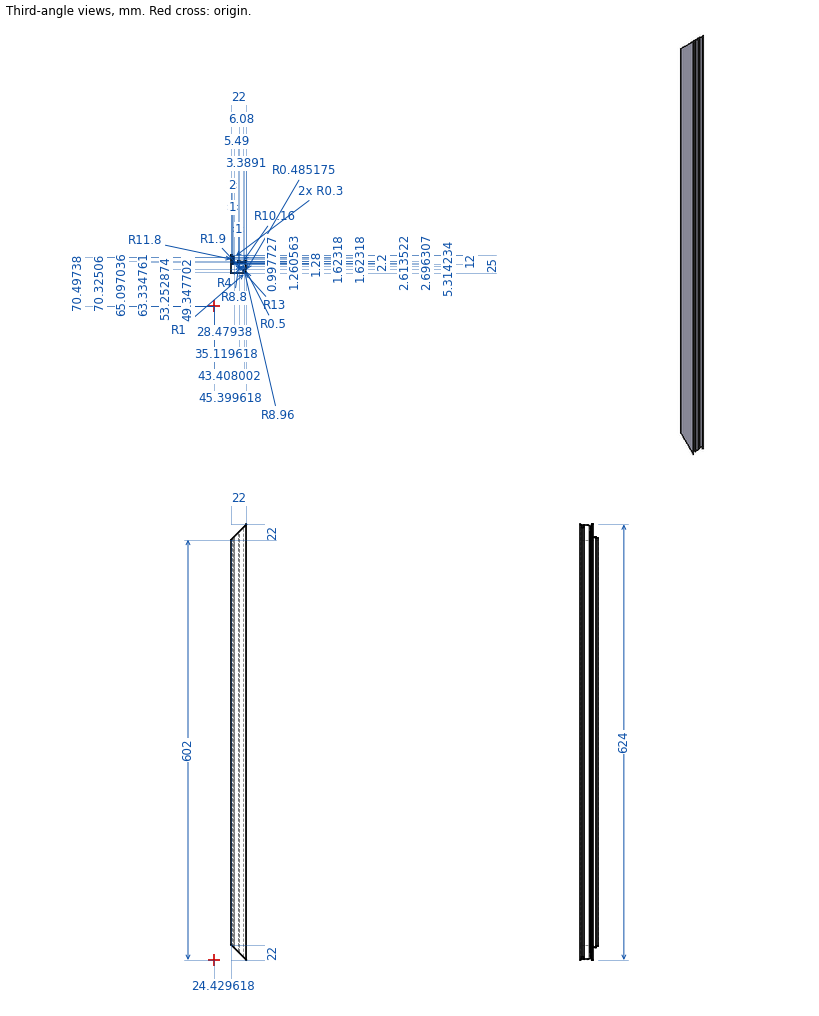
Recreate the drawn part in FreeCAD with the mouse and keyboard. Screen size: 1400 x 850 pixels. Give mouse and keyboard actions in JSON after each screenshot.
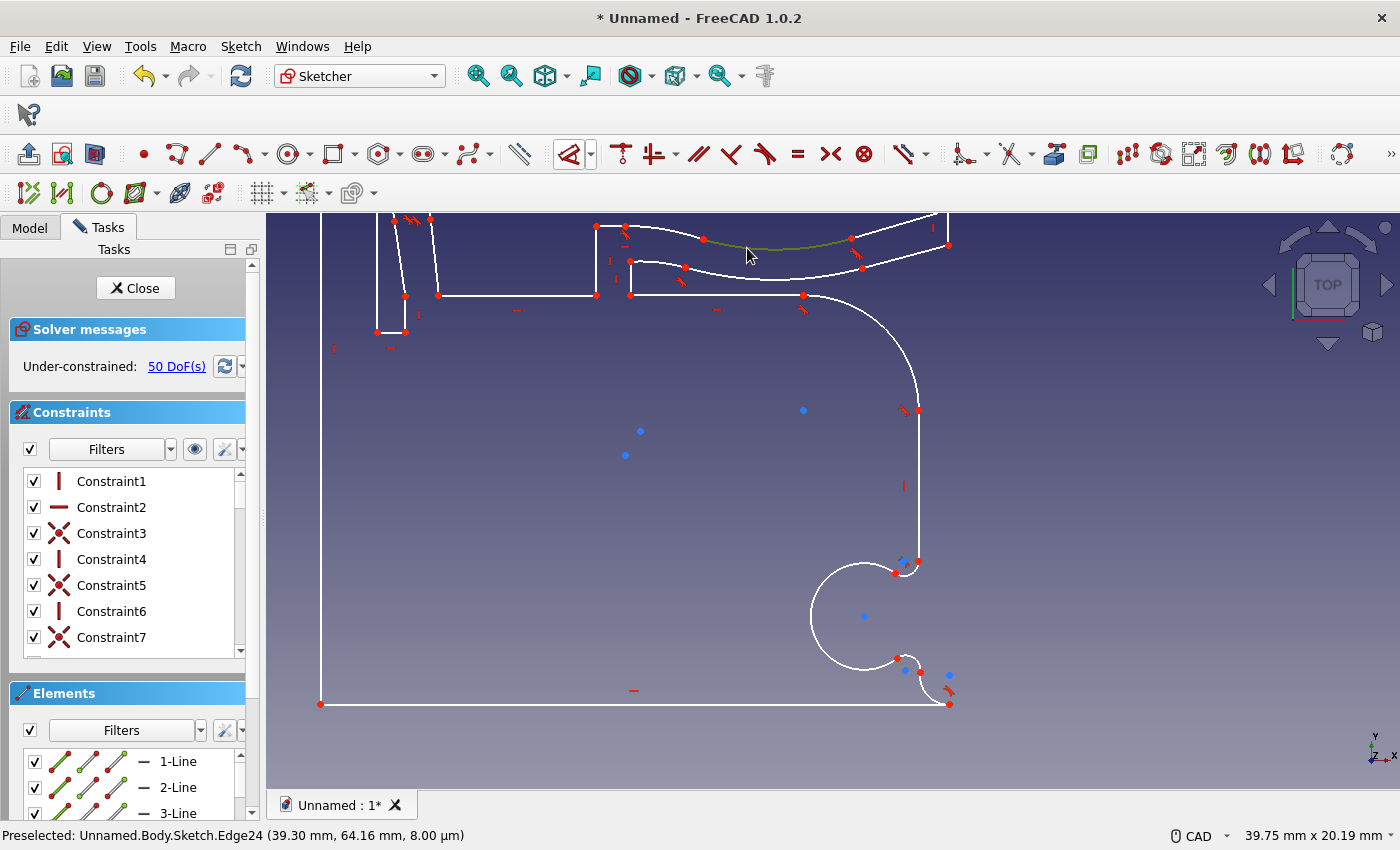
{"action": "scroll", "coordinate": [923, 689], "scroll_direction": "down", "scroll_amount": 3}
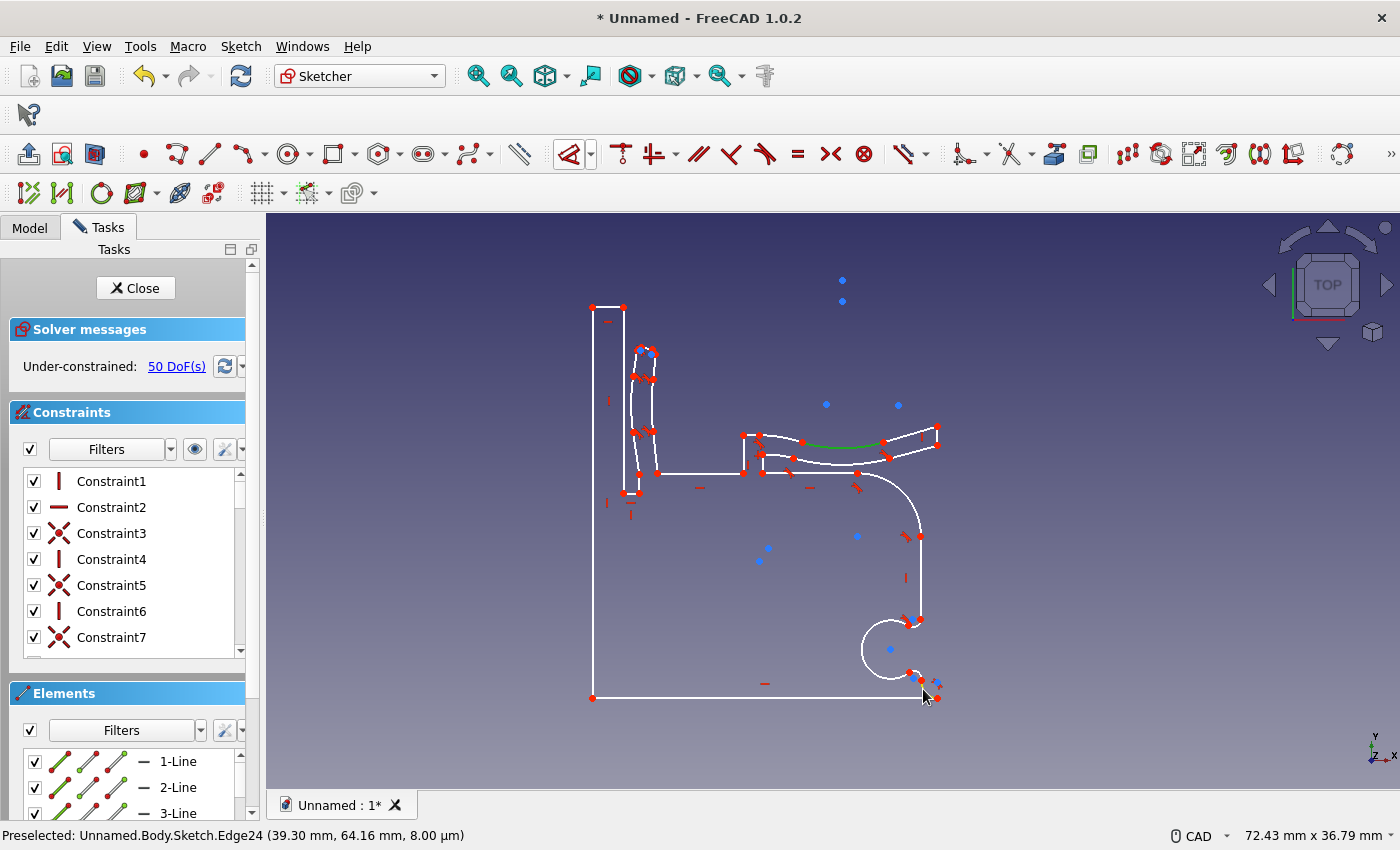
{"action": "left_click", "coordinate": [790, 439]}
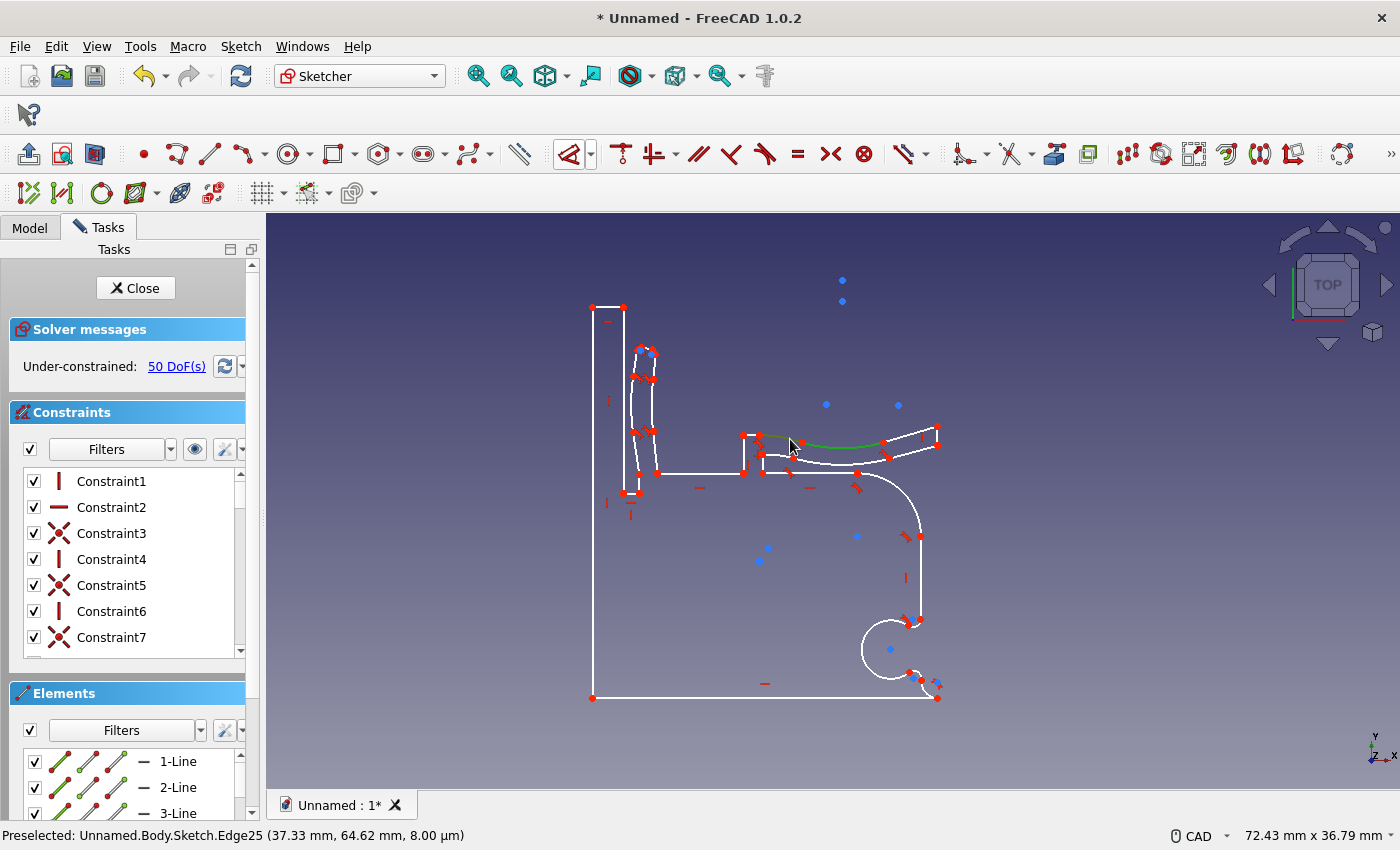
{"action": "key", "text": "t"}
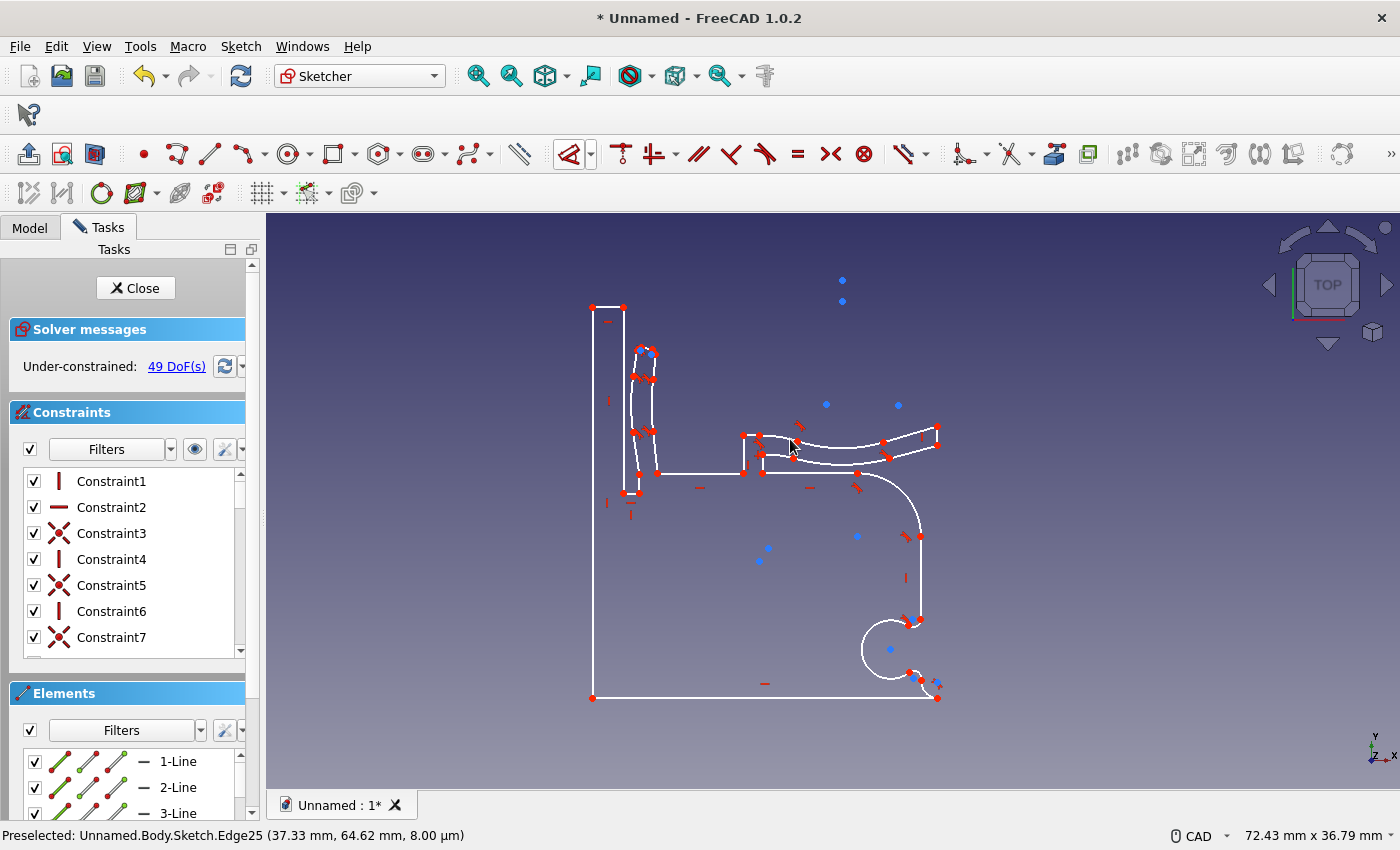
{"action": "scroll", "coordinate": [923, 688], "scroll_direction": "up", "scroll_amount": 3}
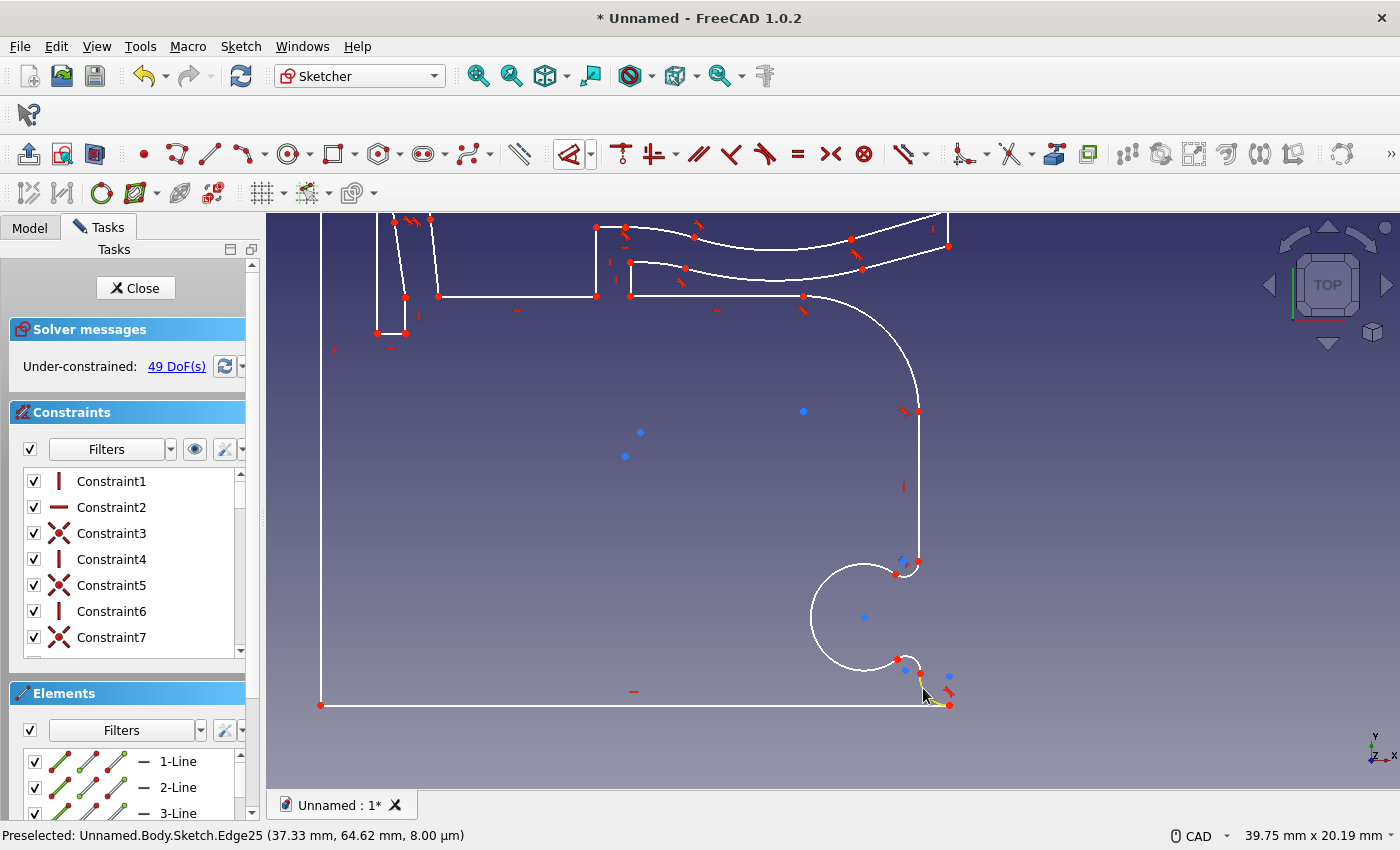
{"action": "left_click", "coordinate": [922, 688]}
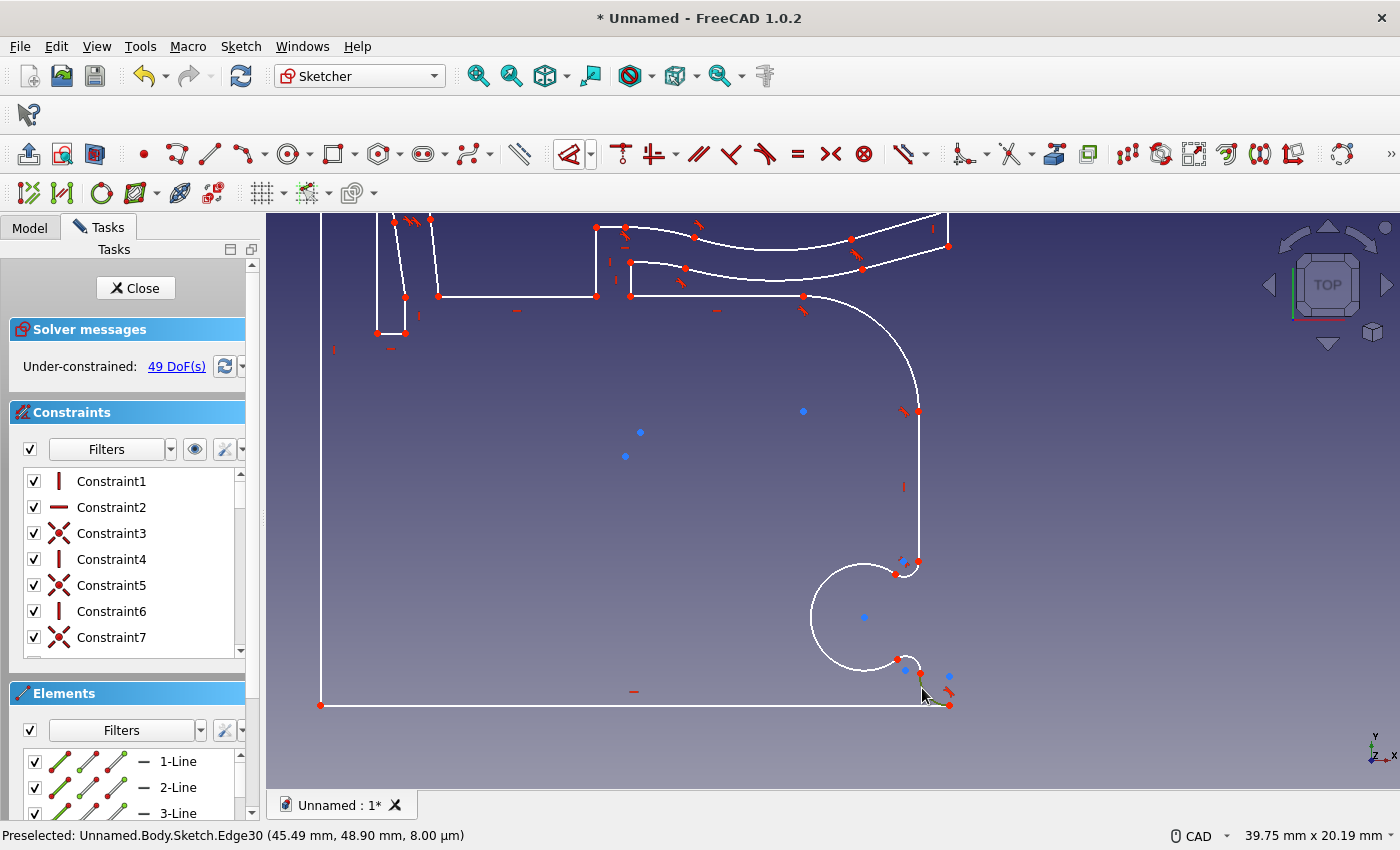
{"action": "scroll", "coordinate": [918, 664], "scroll_direction": "up", "scroll_amount": 2}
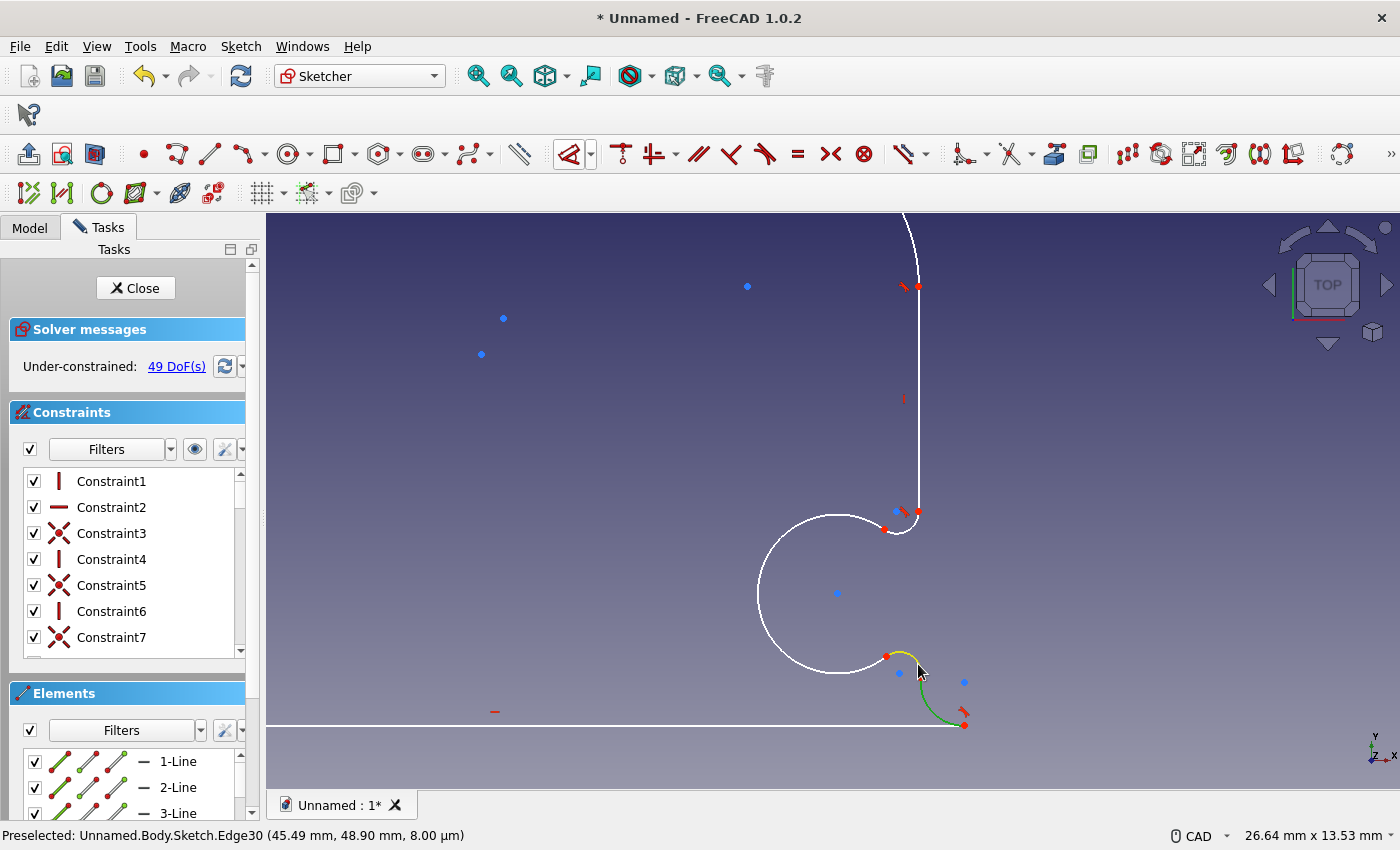
{"action": "left_click", "coordinate": [918, 663]}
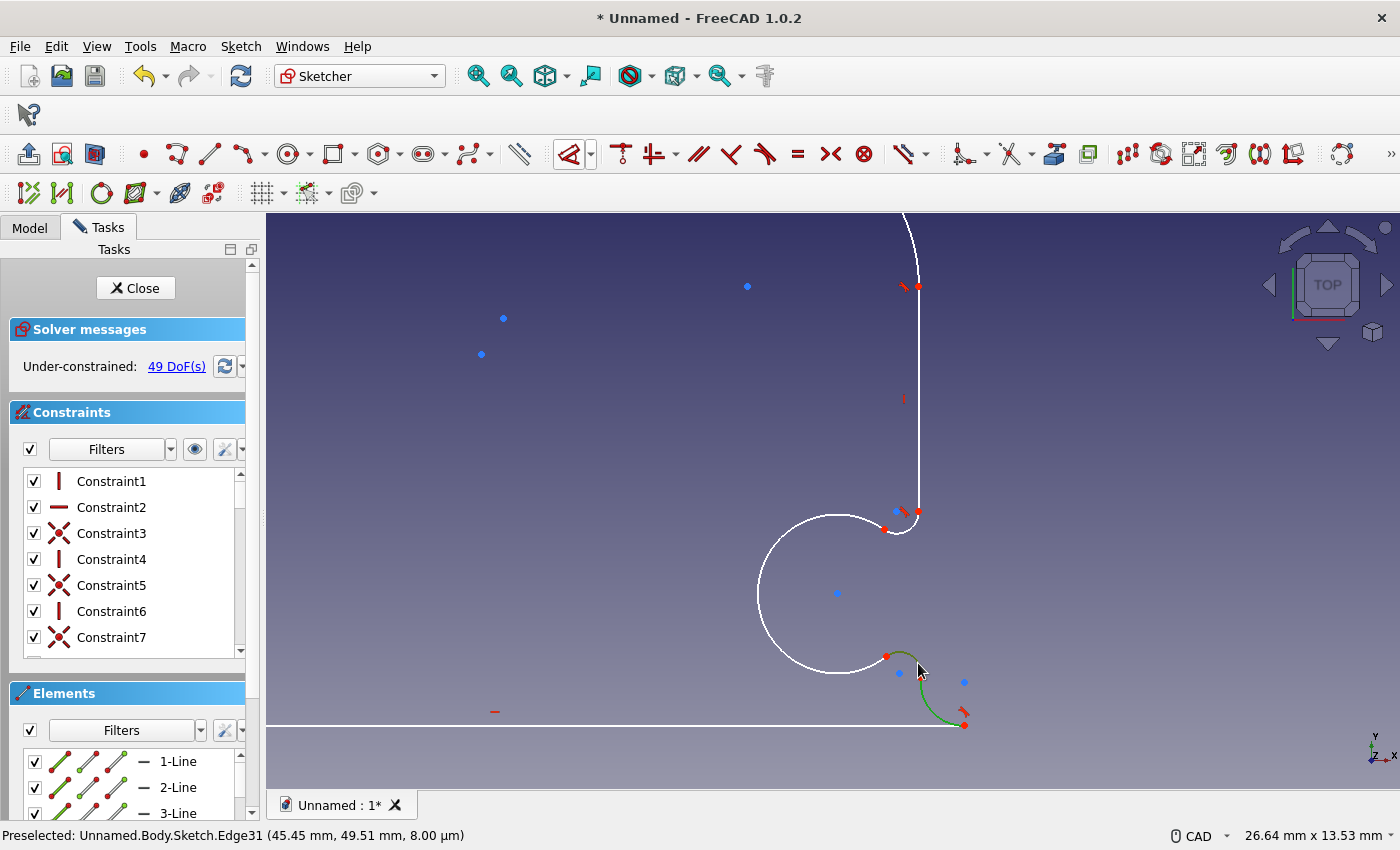
{"action": "key", "text": "t"}